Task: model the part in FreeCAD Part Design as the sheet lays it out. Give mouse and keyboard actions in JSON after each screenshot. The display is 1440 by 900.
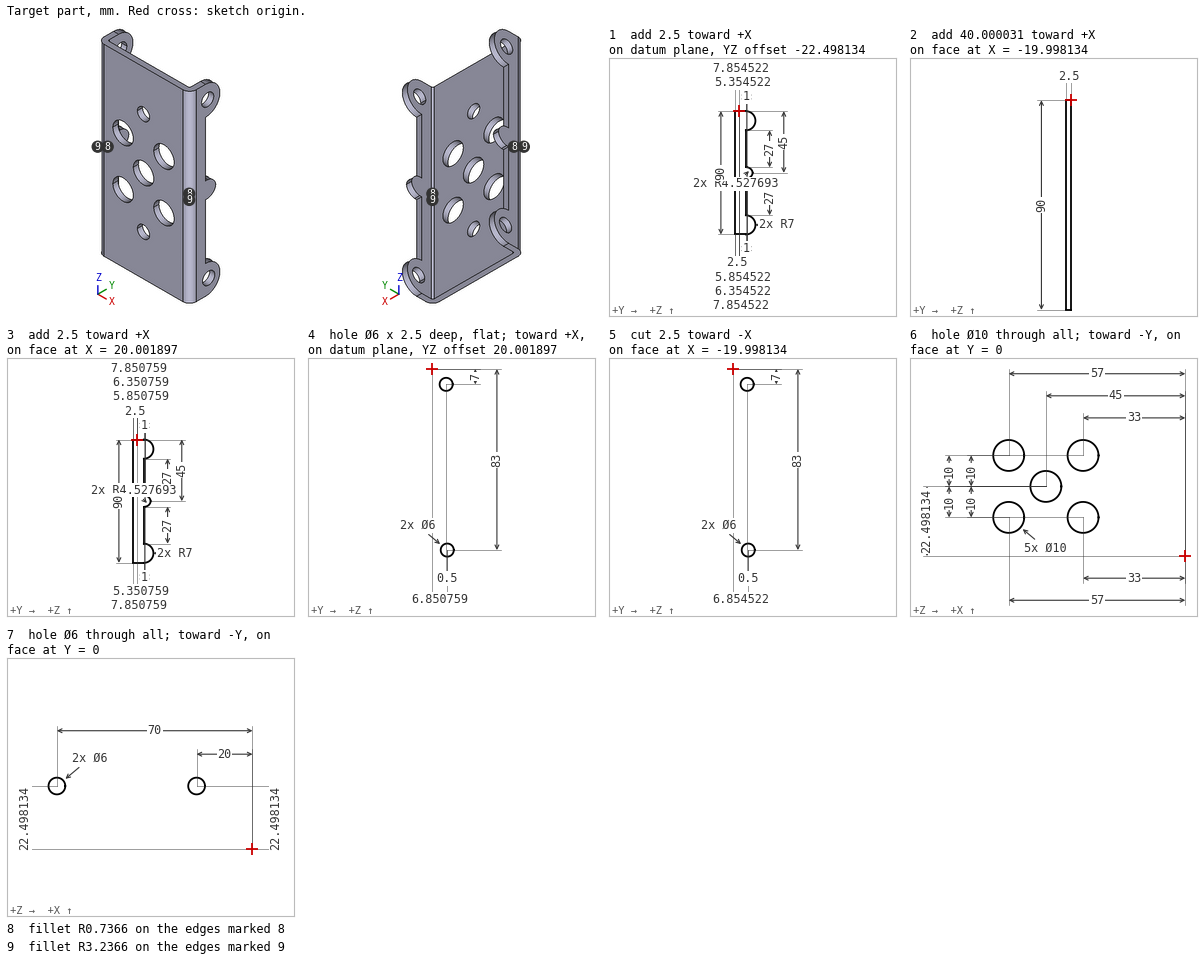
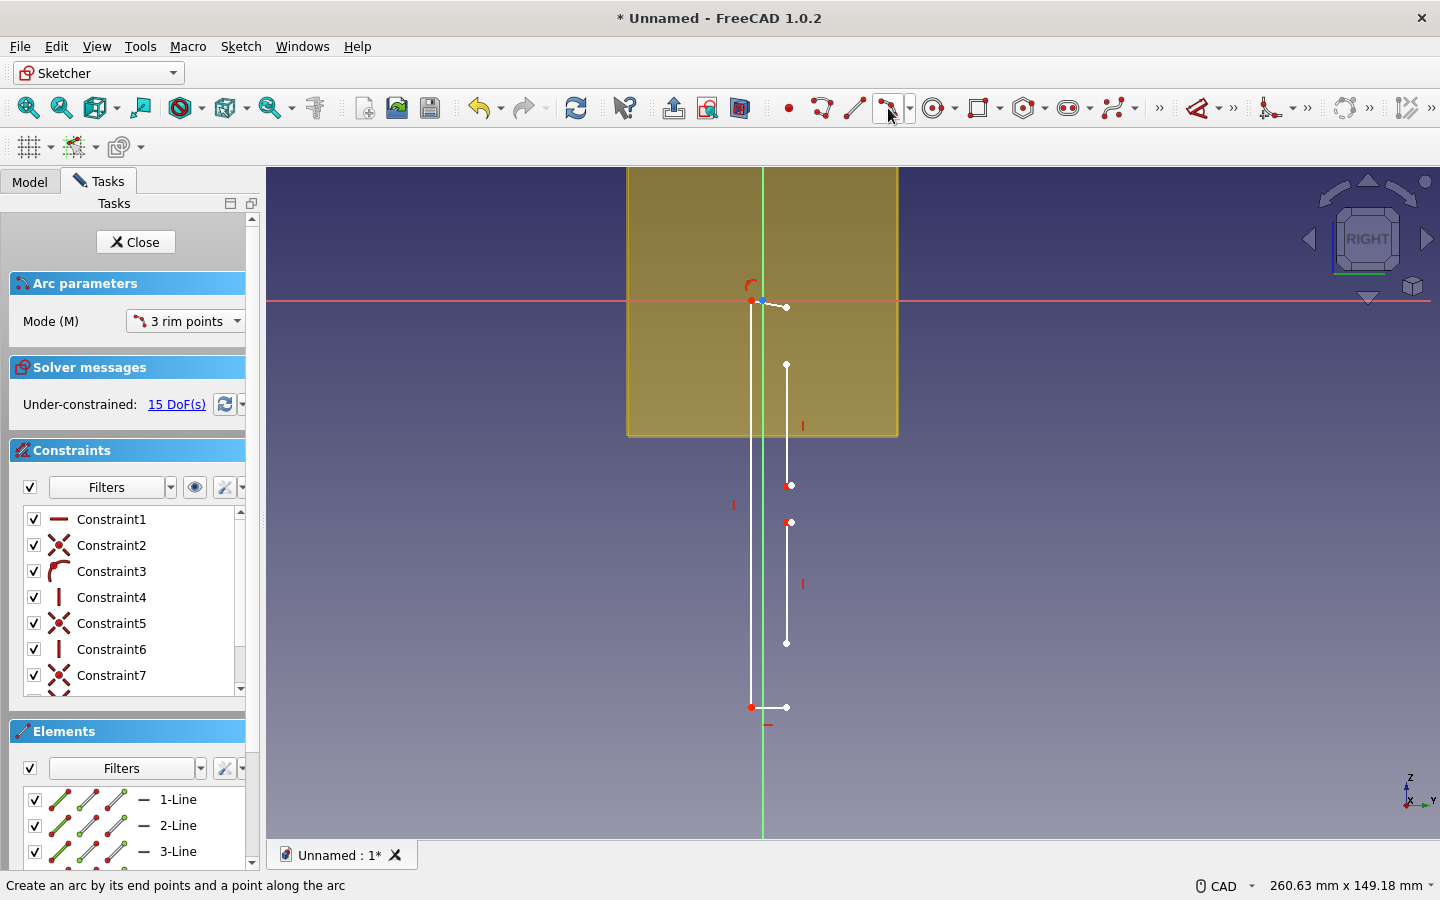
{"action": "left_click", "coordinate": [787, 307]}
{"action": "left_click", "coordinate": [787, 364]}
{"action": "left_click", "coordinate": [818, 332]}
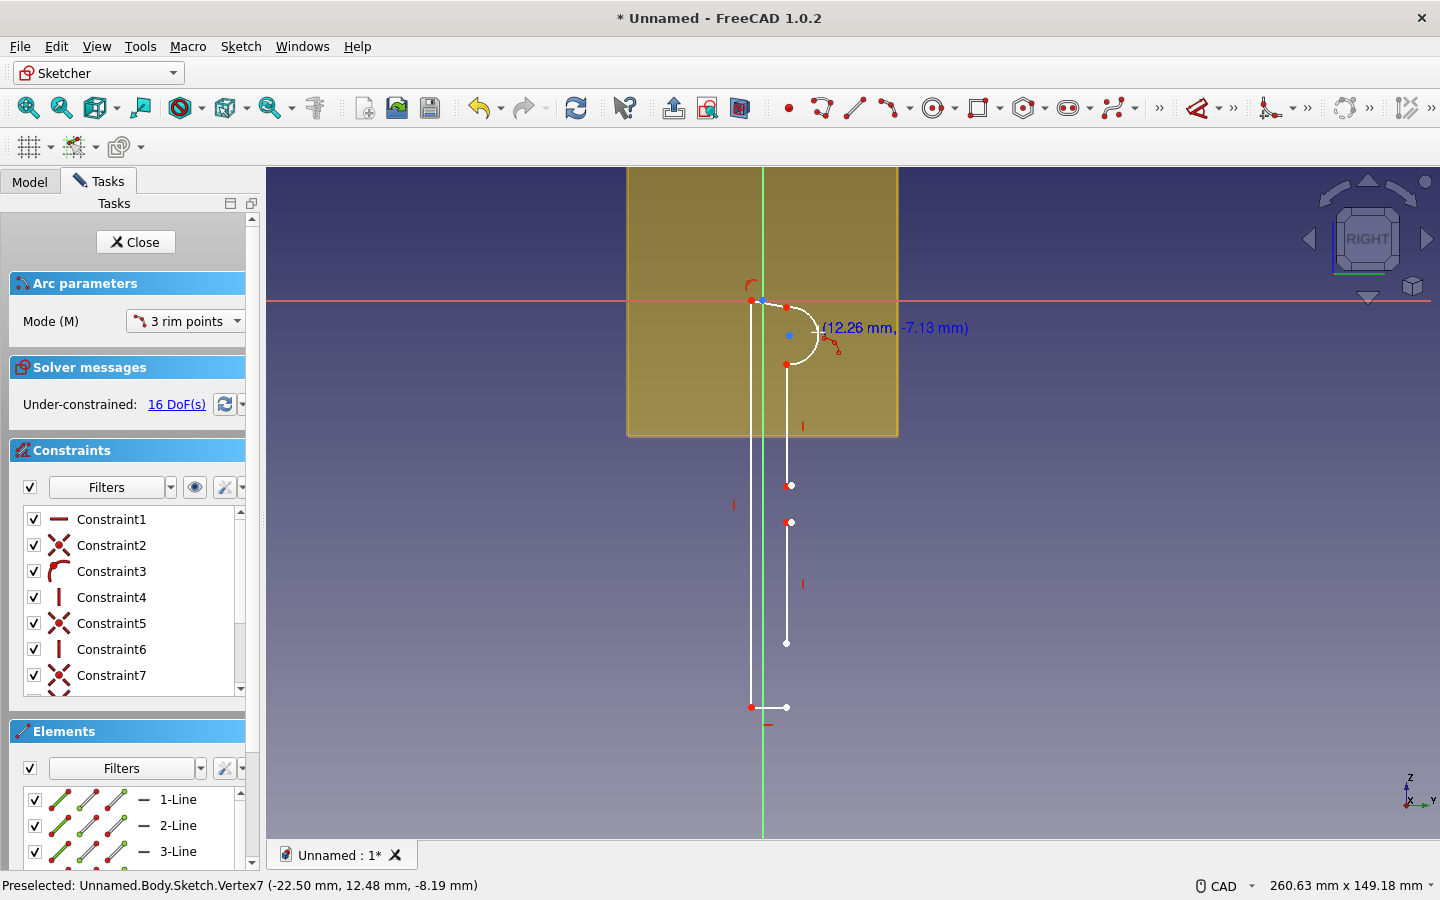
{"action": "scroll", "coordinate": [791, 486], "scroll_direction": "up", "scroll_amount": 10}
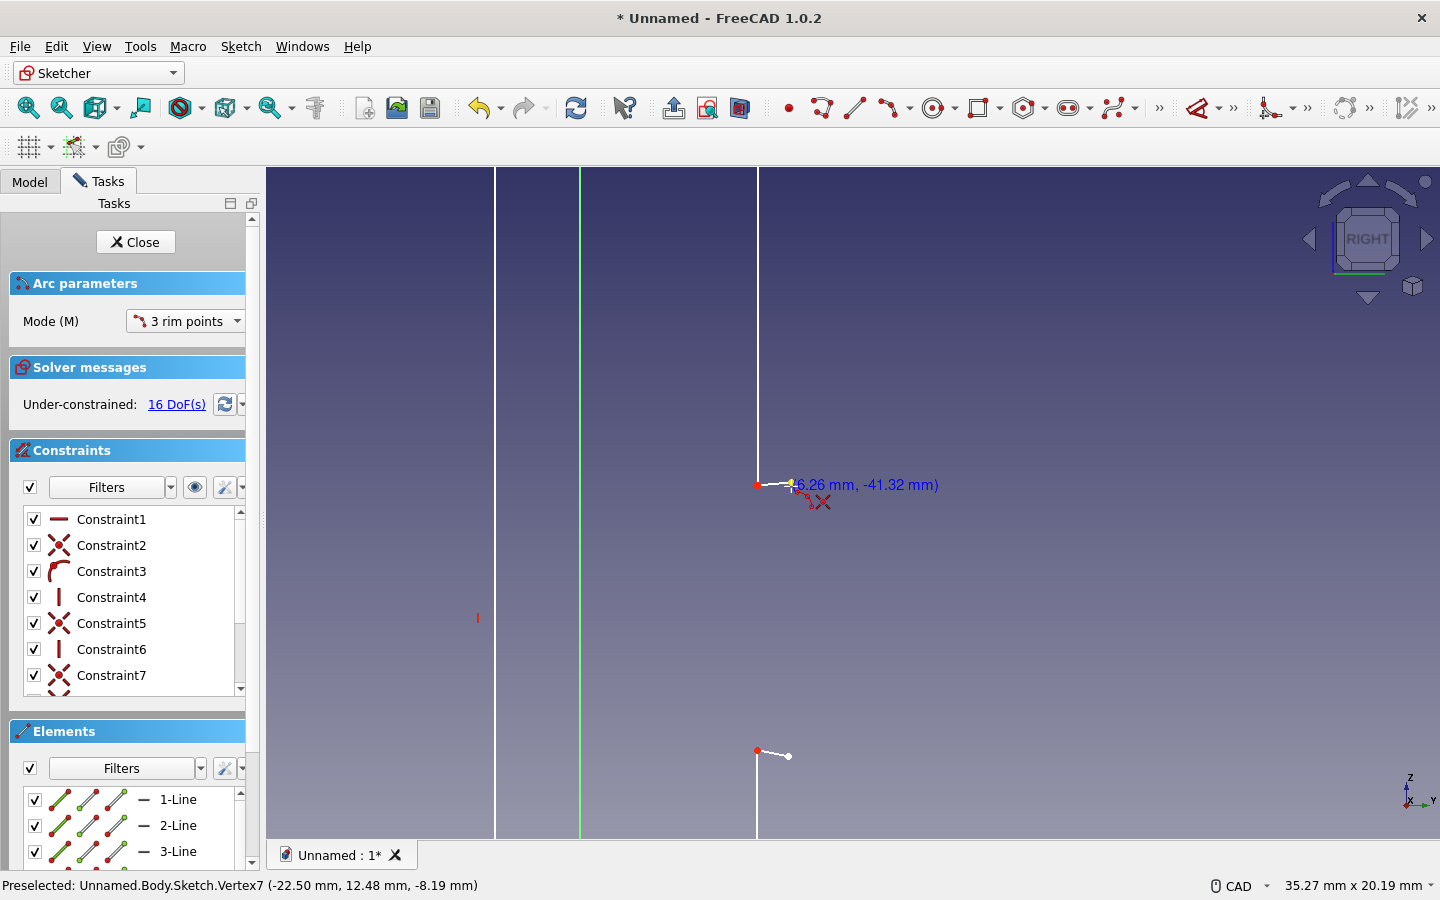
{"action": "left_click", "coordinate": [792, 482]}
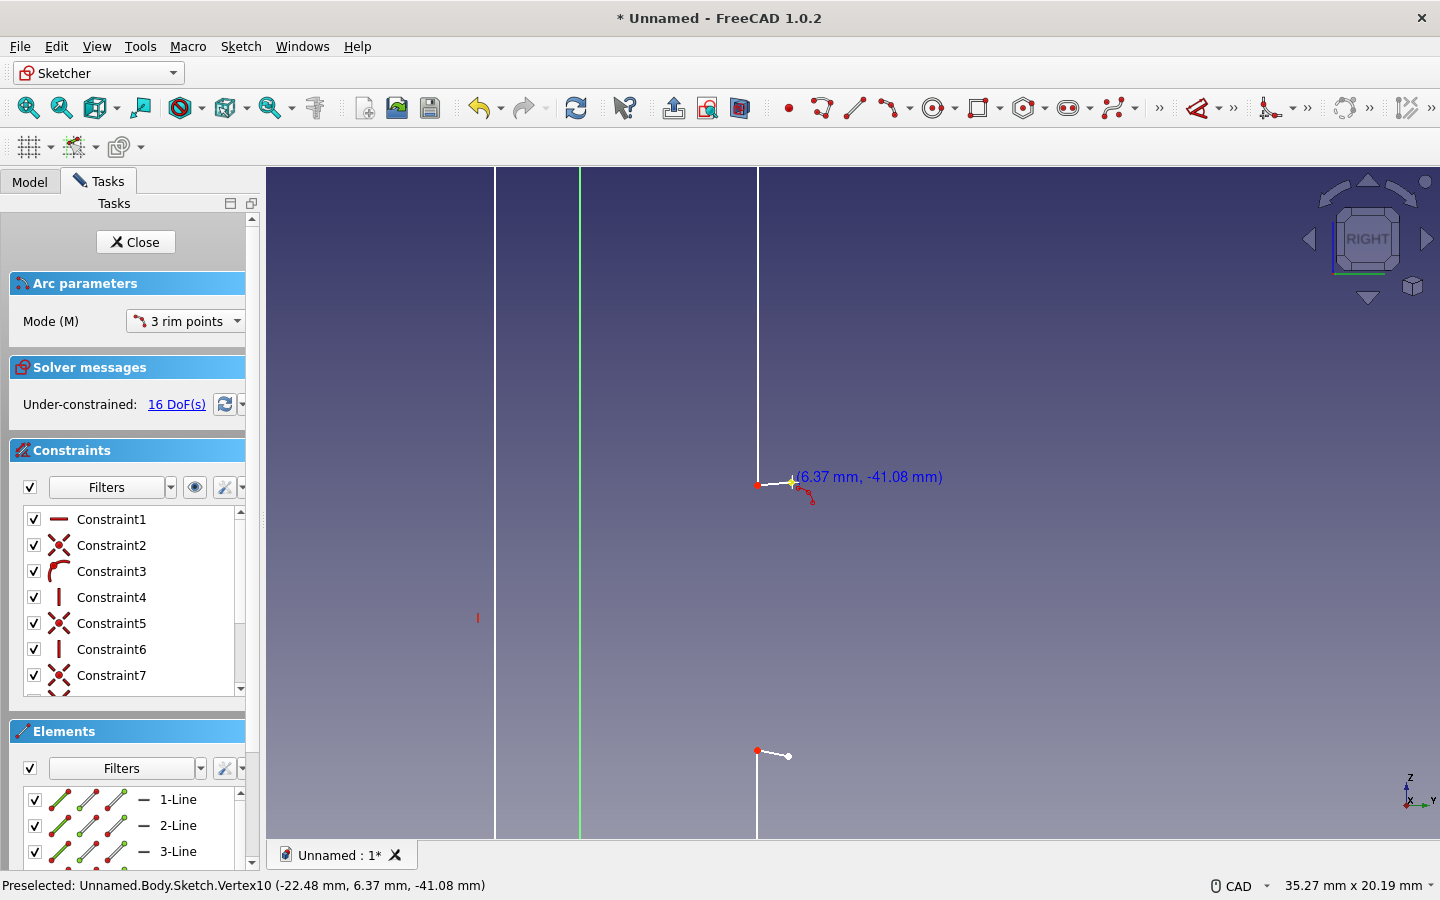
{"action": "scroll", "coordinate": [791, 486], "scroll_direction": "down", "scroll_amount": 10}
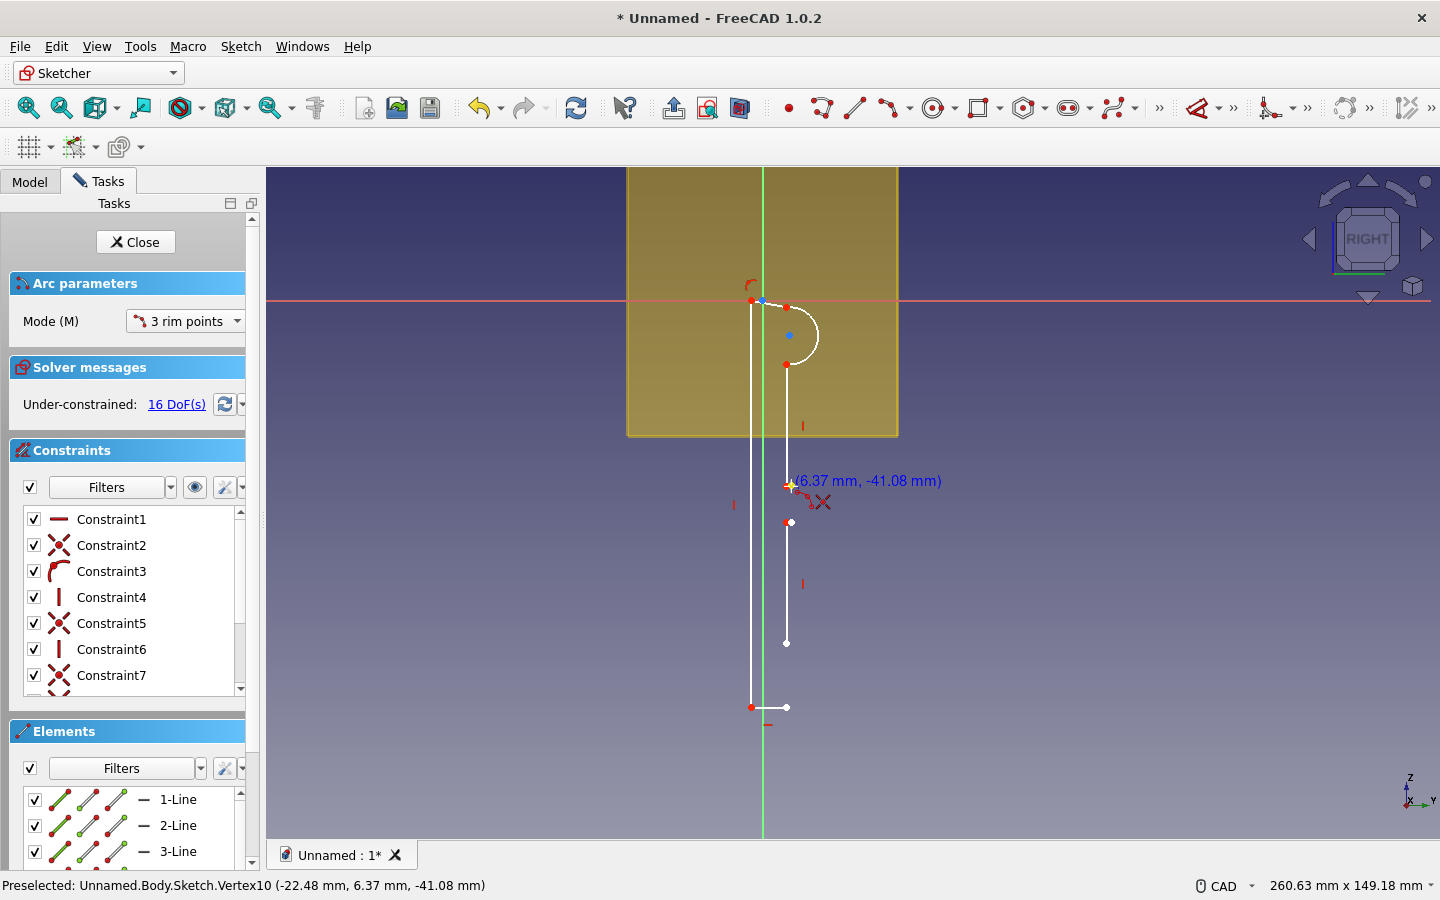
{"action": "left_click", "coordinate": [809, 504]}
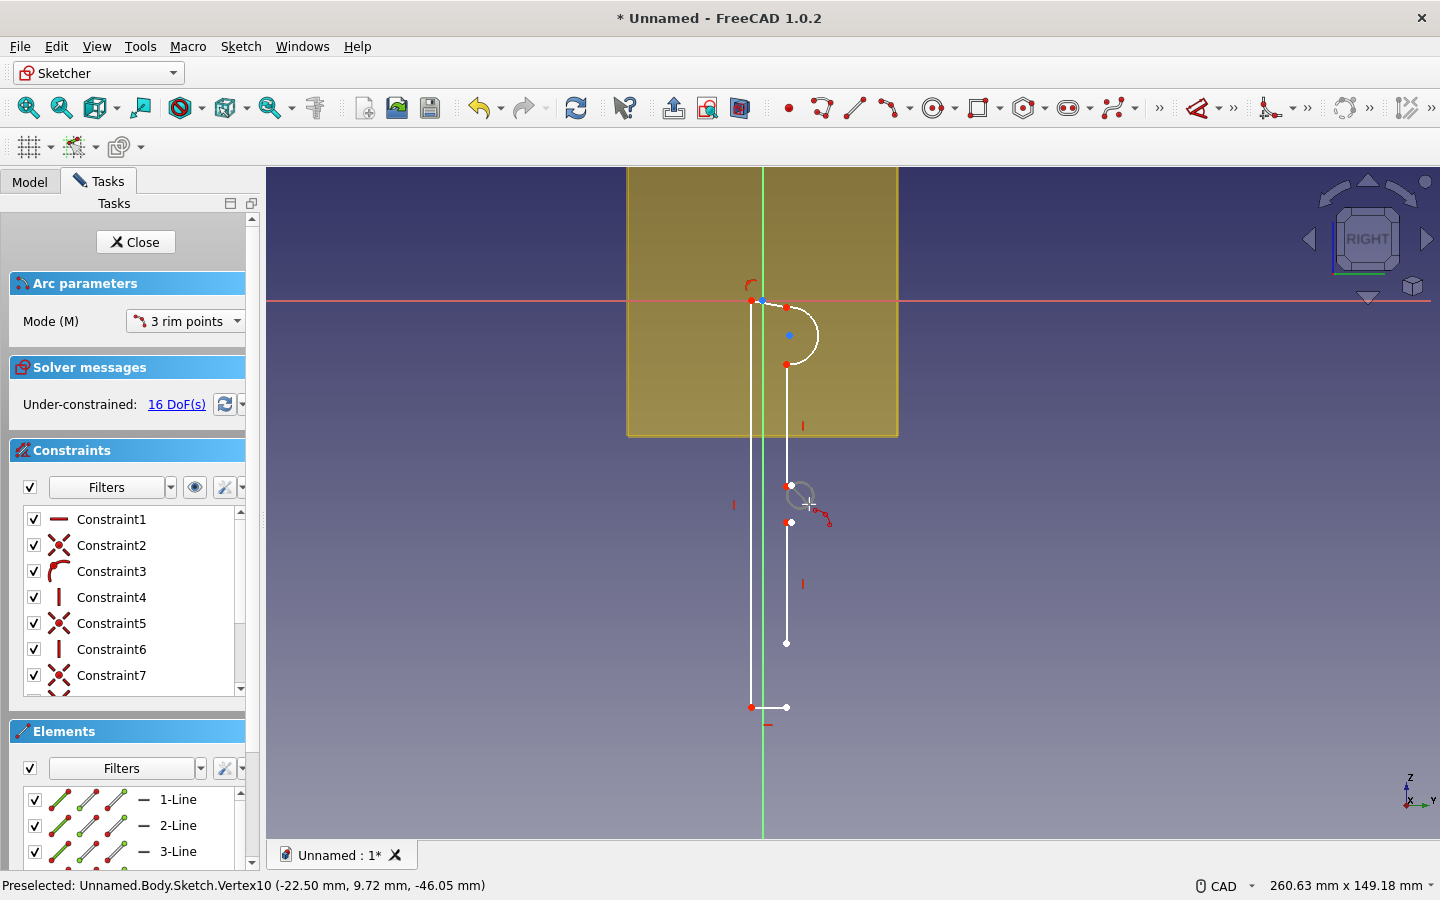
{"action": "scroll", "coordinate": [804, 491], "scroll_direction": "up", "scroll_amount": 7}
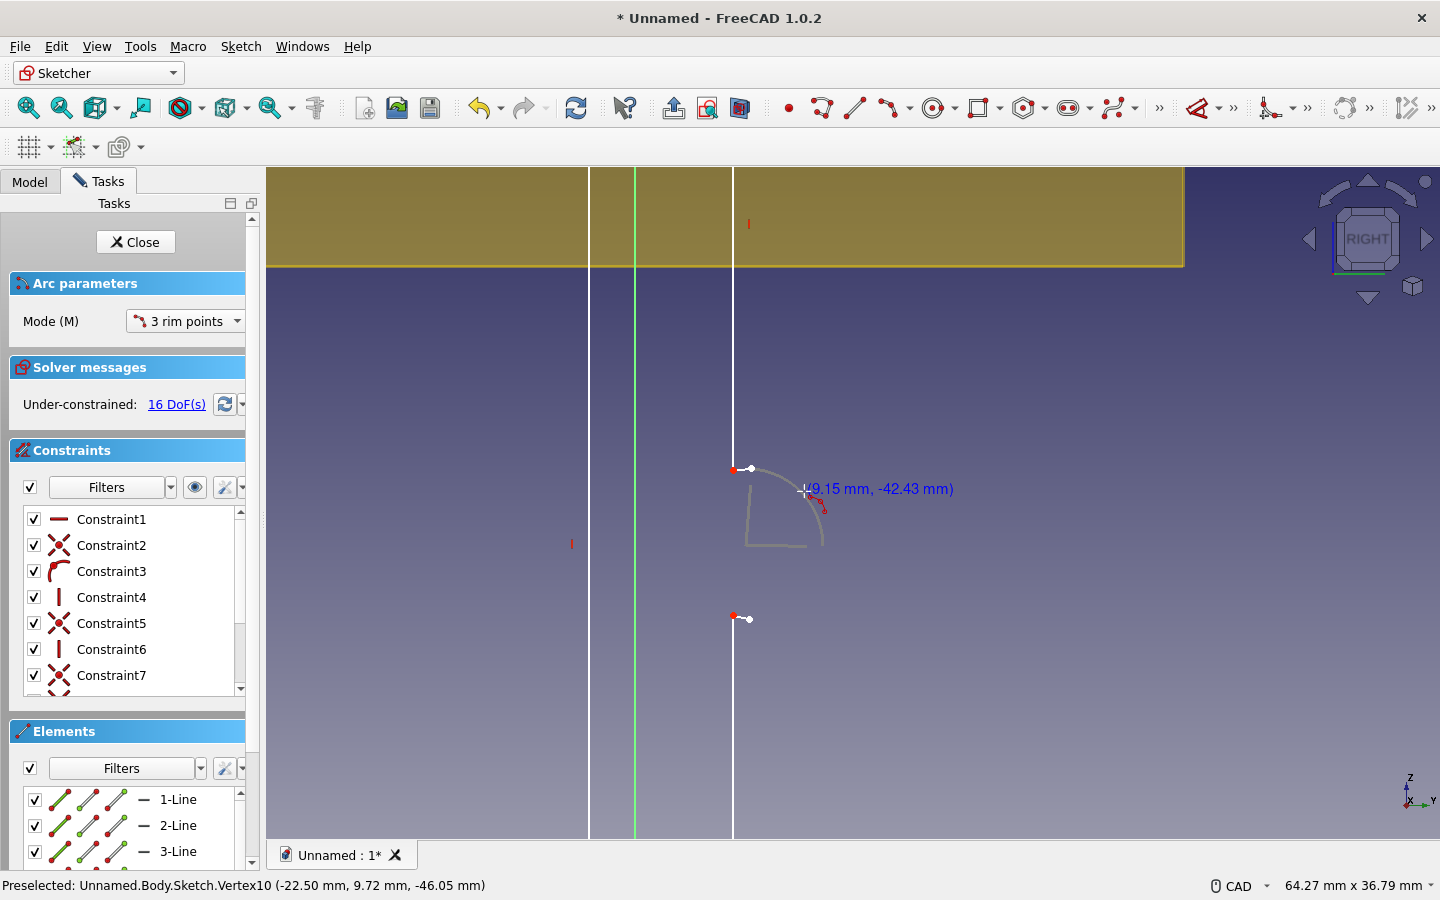
{"action": "left_click", "coordinate": [801, 491]}